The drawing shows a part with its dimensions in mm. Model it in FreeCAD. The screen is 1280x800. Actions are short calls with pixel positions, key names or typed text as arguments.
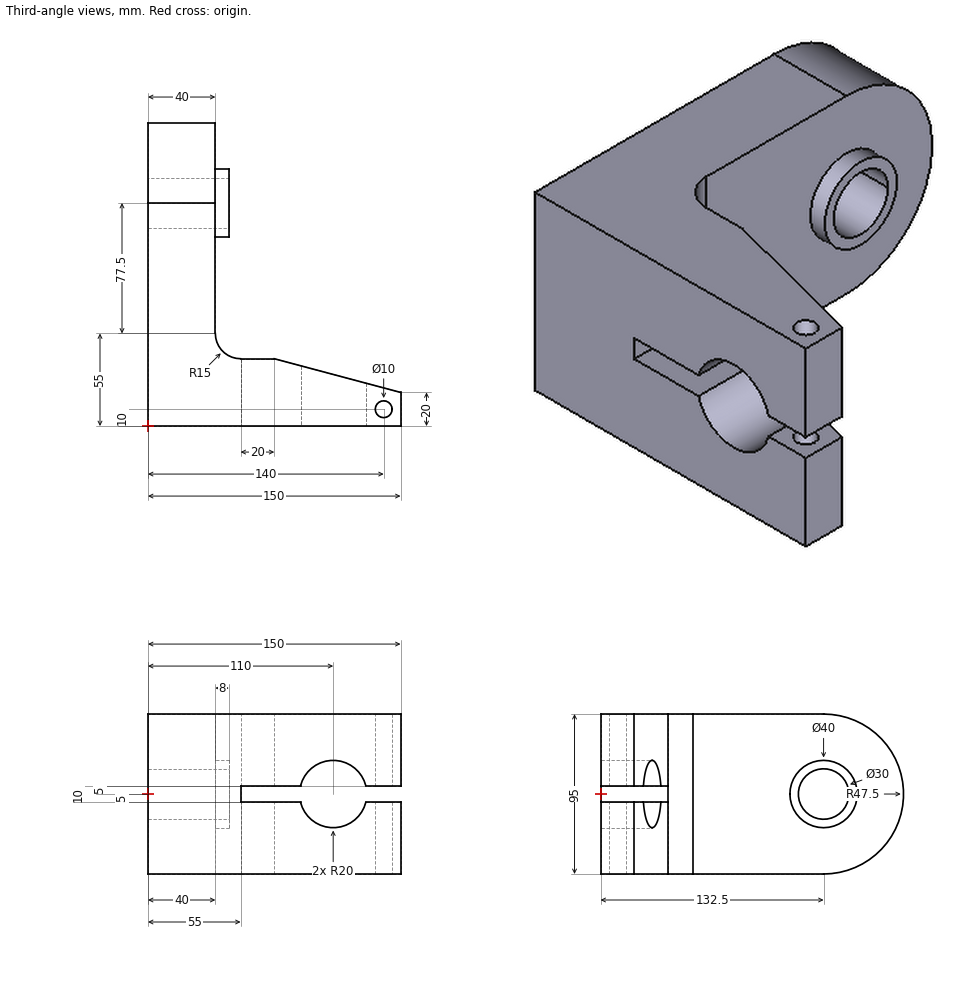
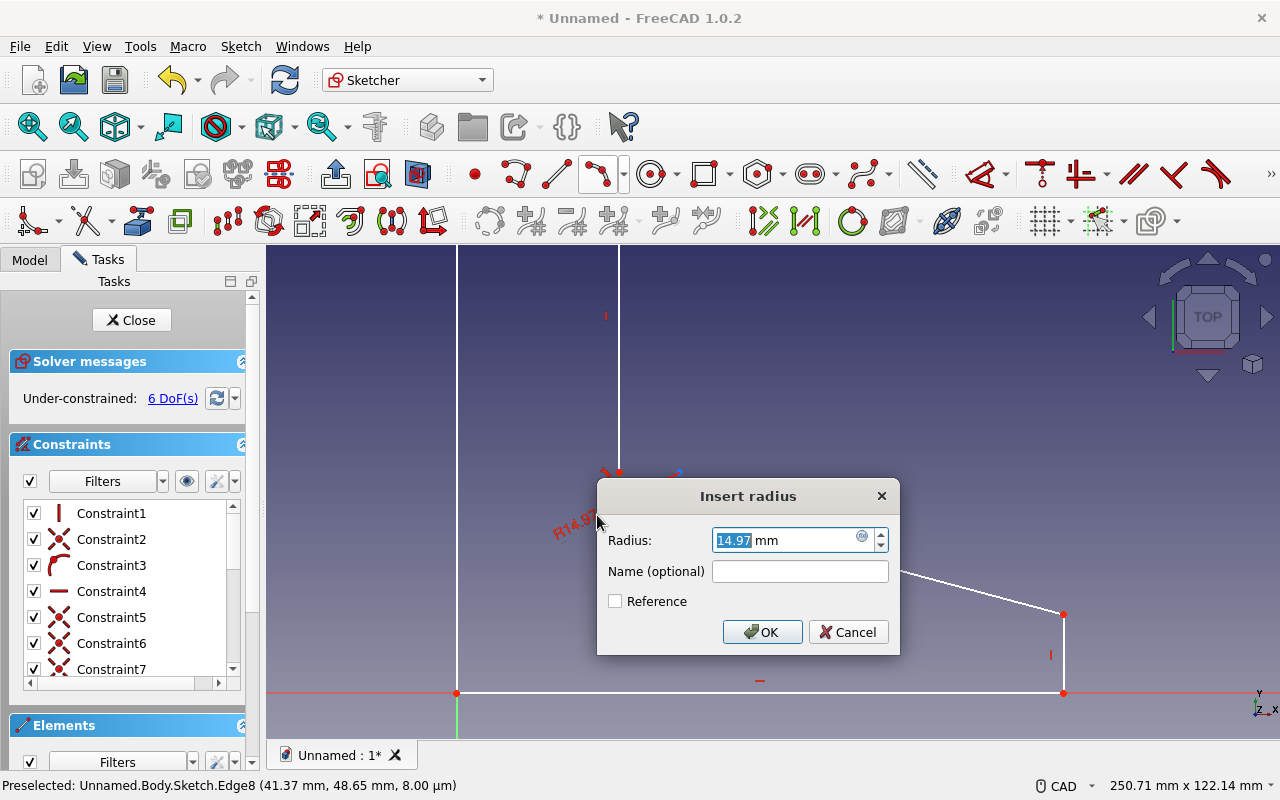
text(15)
key(Return)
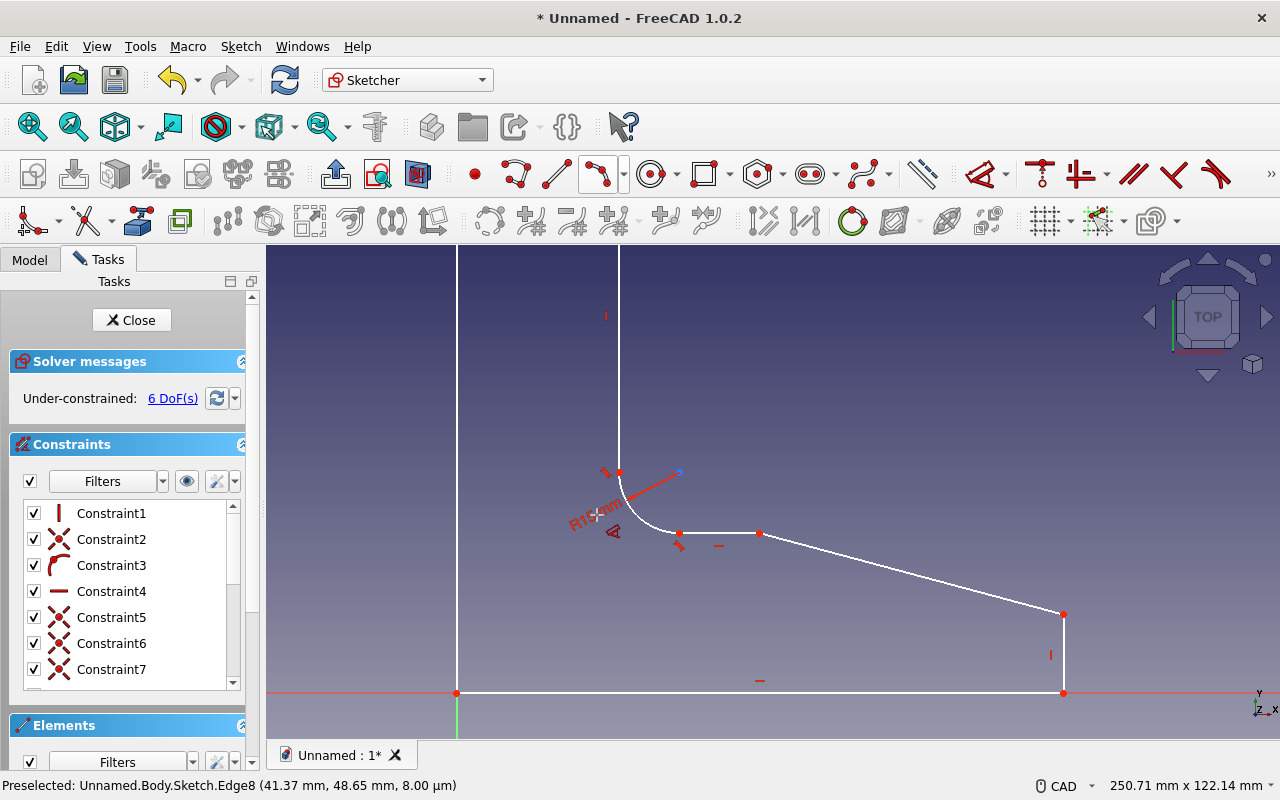
scroll(637, 573, down, 3)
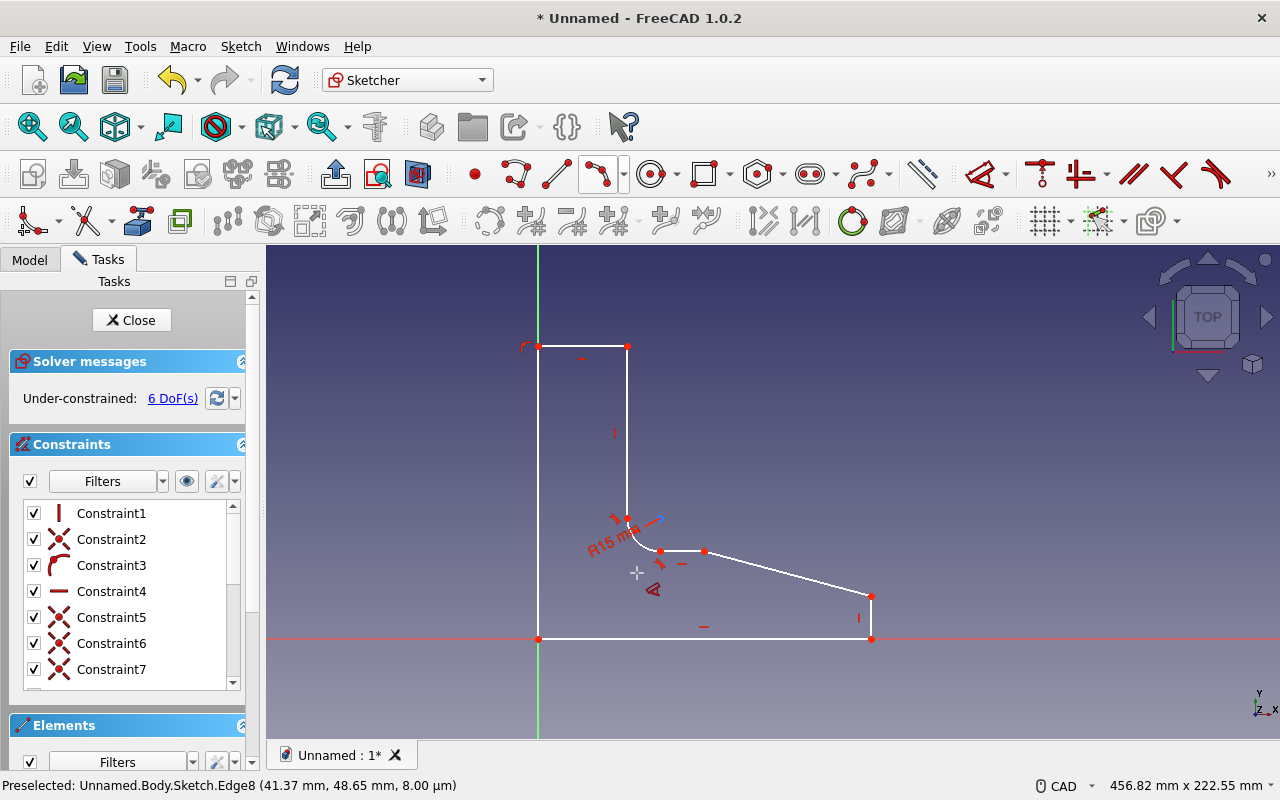
click(601, 346)
click(583, 312)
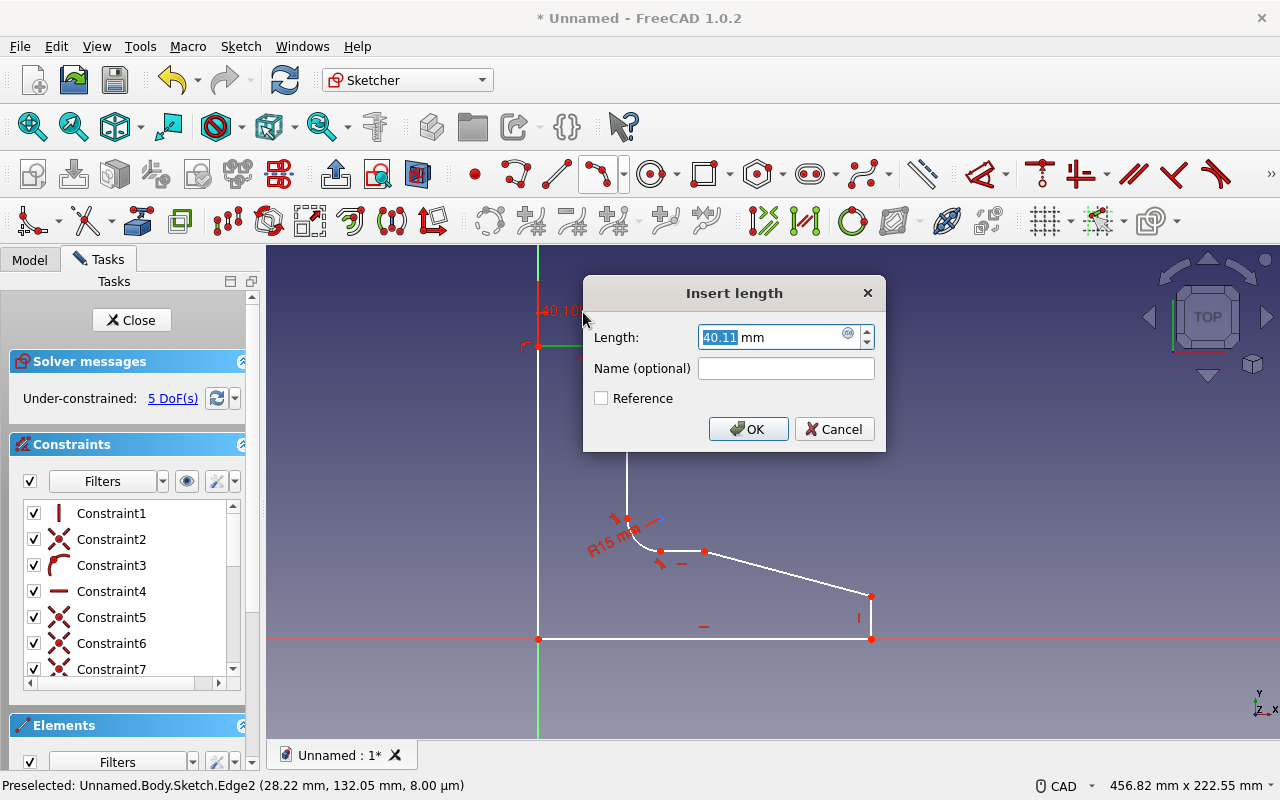
text(40)
key(Return)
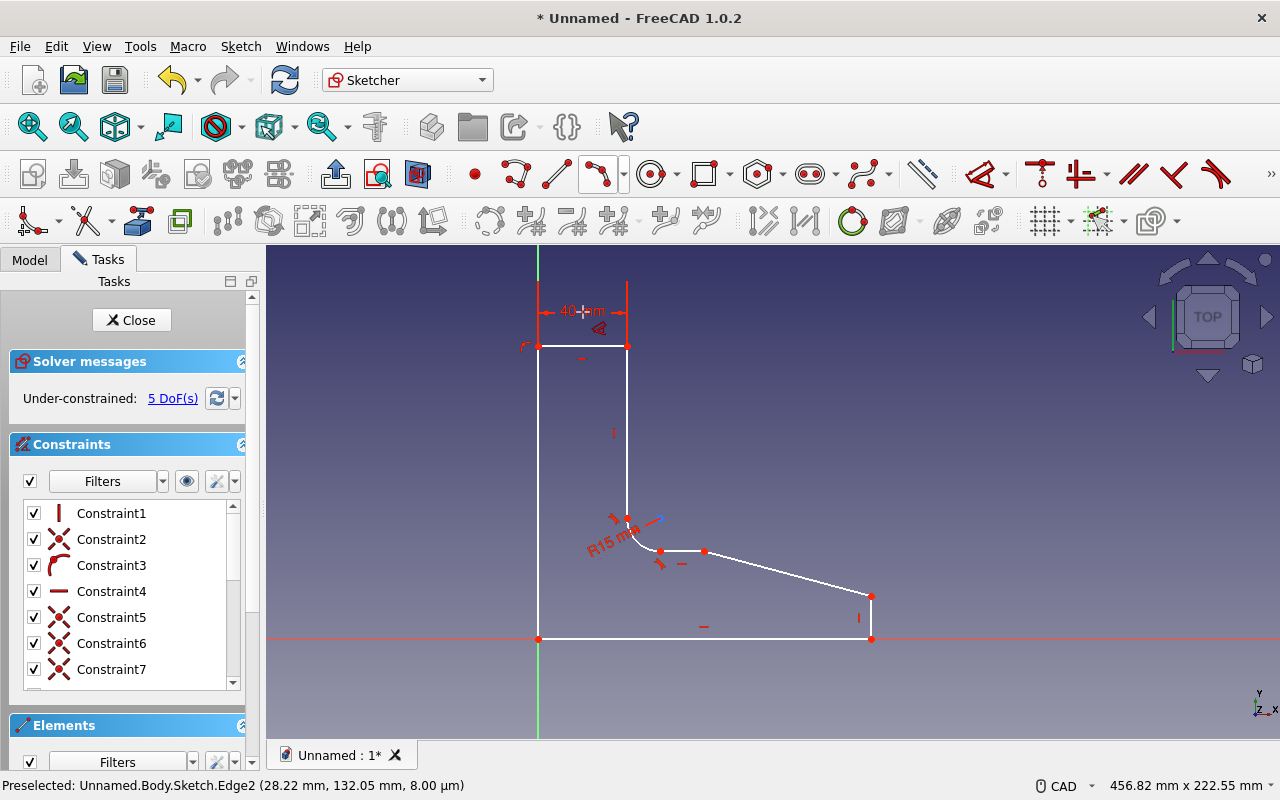
click(871, 626)
click(905, 618)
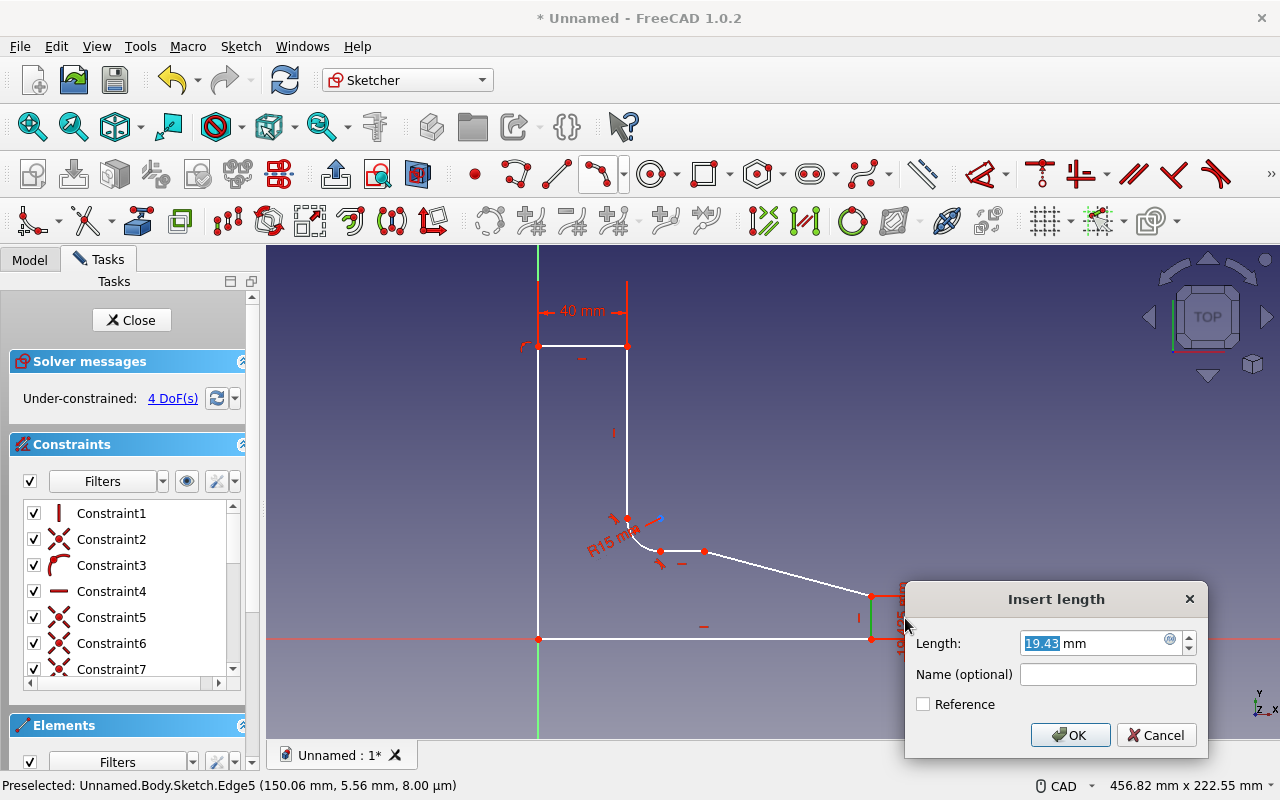
text(20)
key(Return)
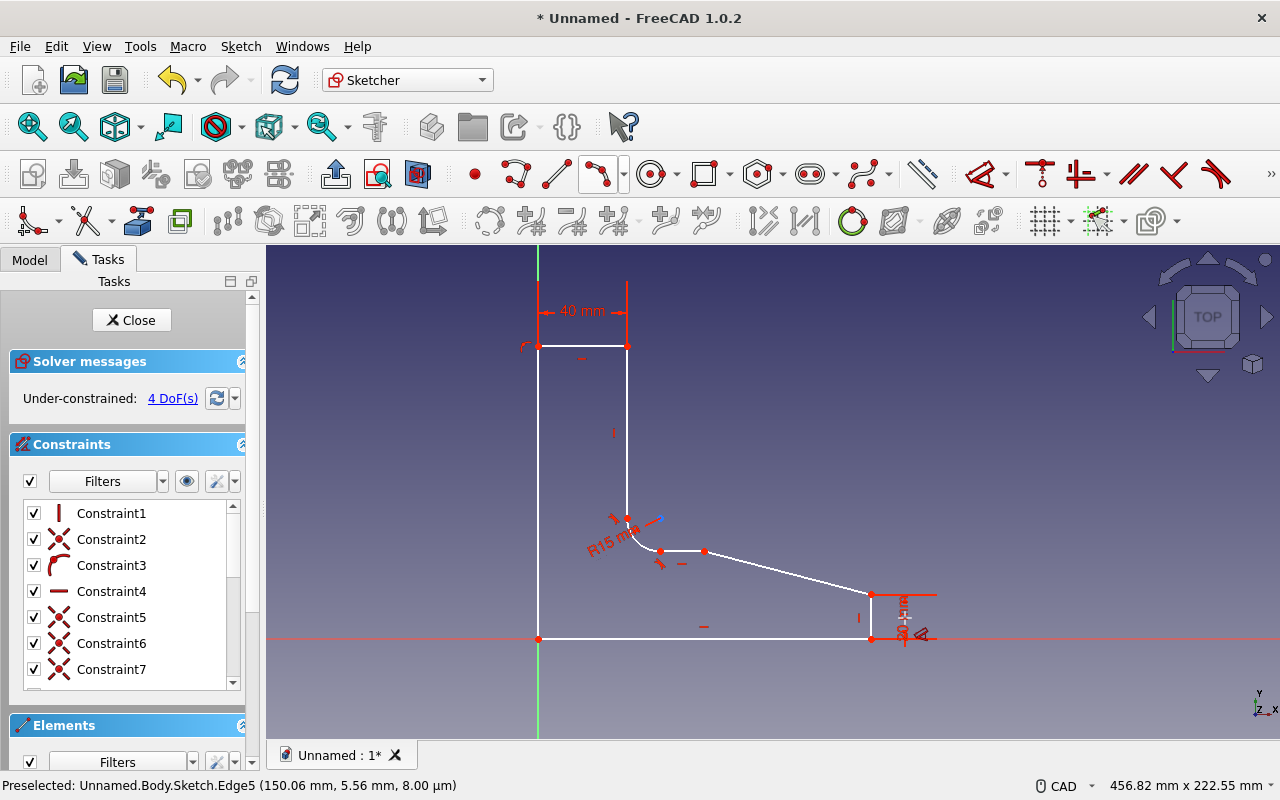
click(691, 551)
click(682, 585)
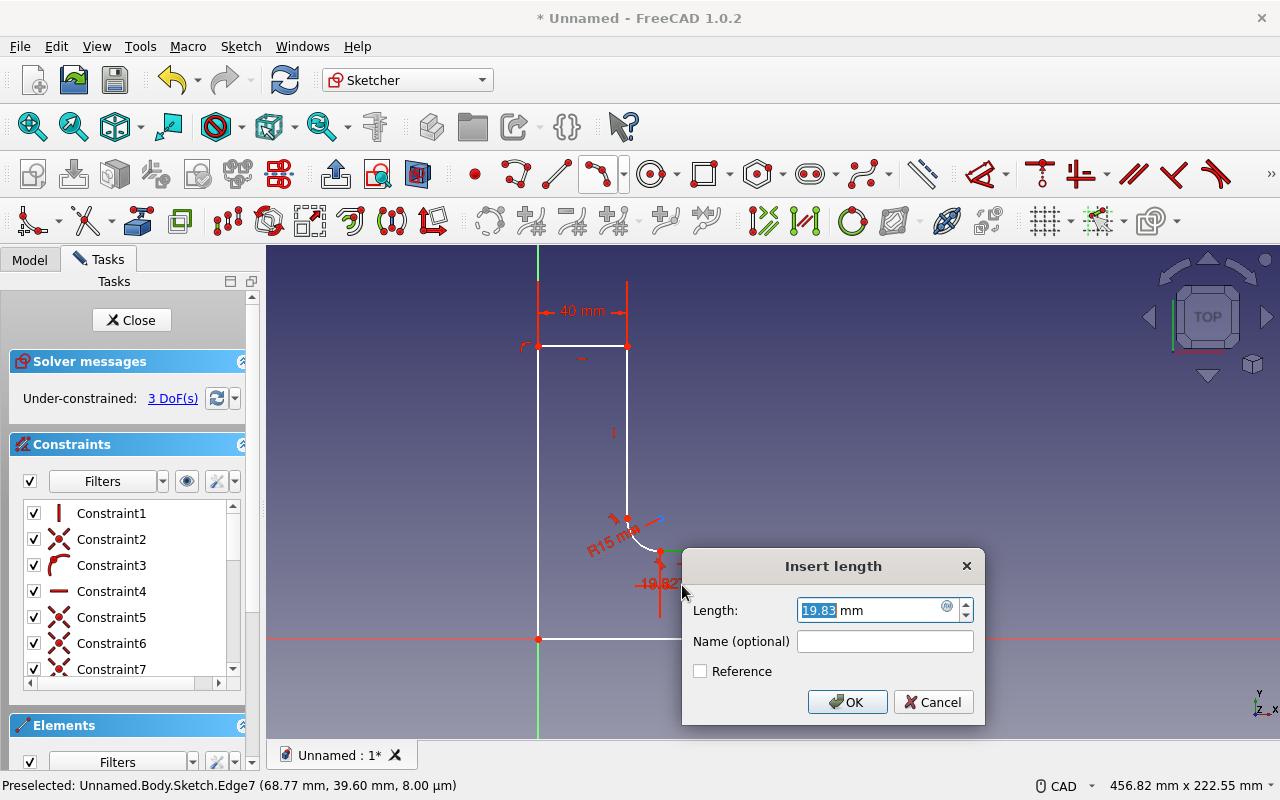
text(20)
key(Return)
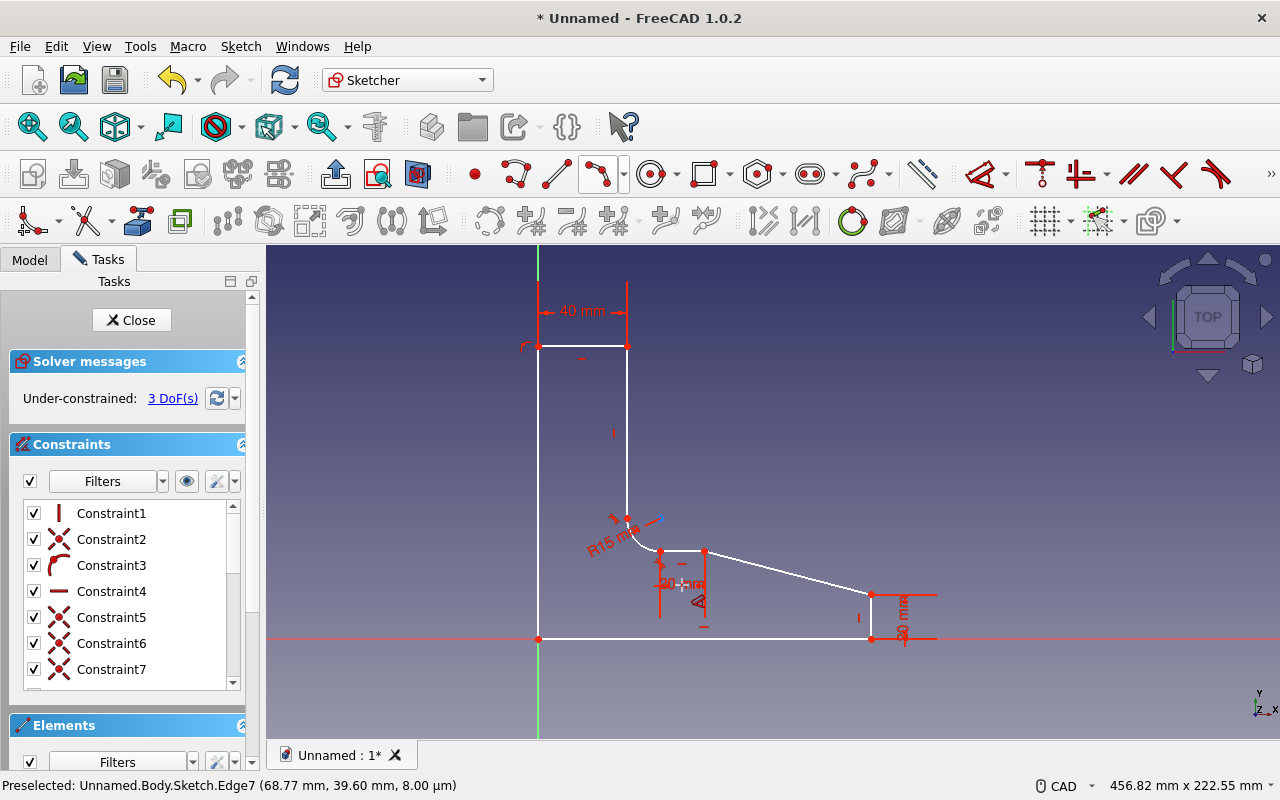
click(638, 639)
click(705, 673)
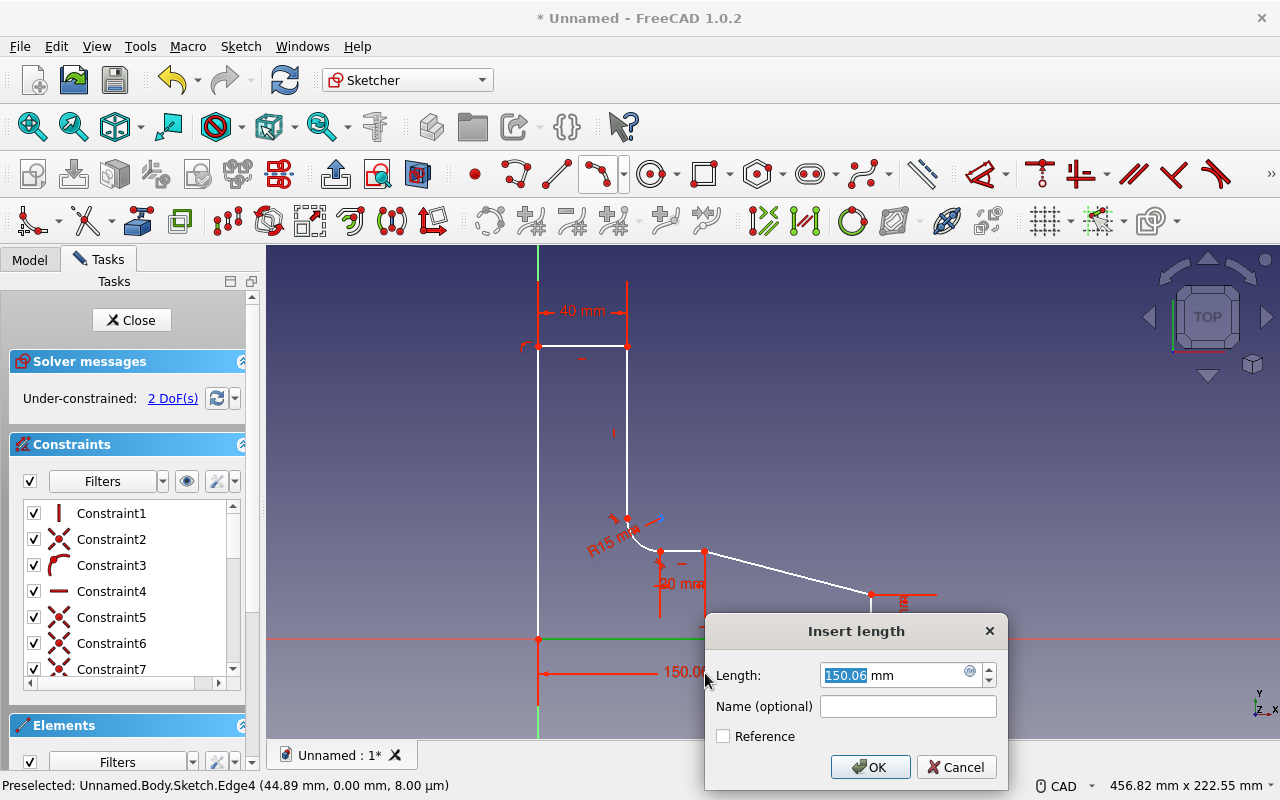
text(150)
key(Return)